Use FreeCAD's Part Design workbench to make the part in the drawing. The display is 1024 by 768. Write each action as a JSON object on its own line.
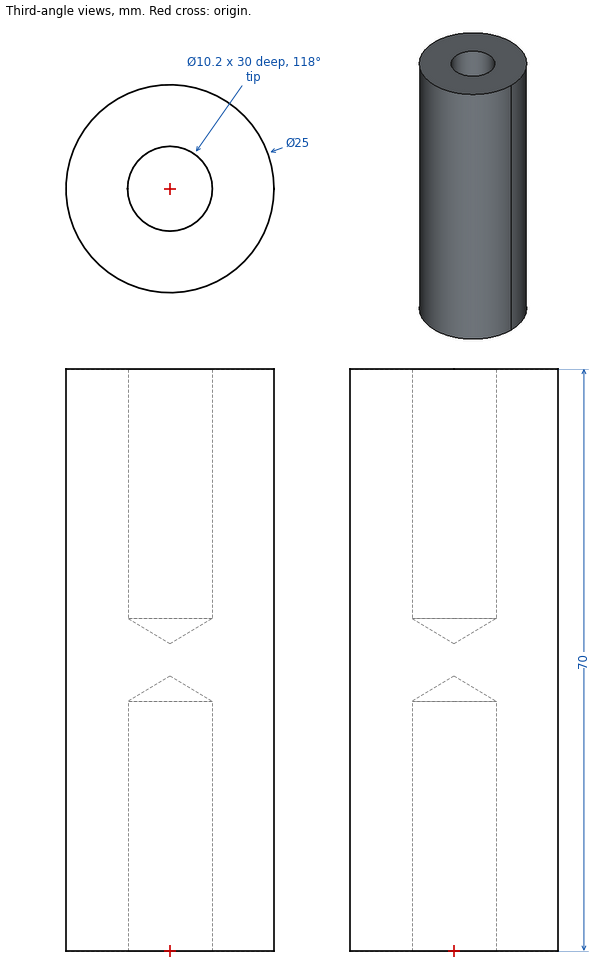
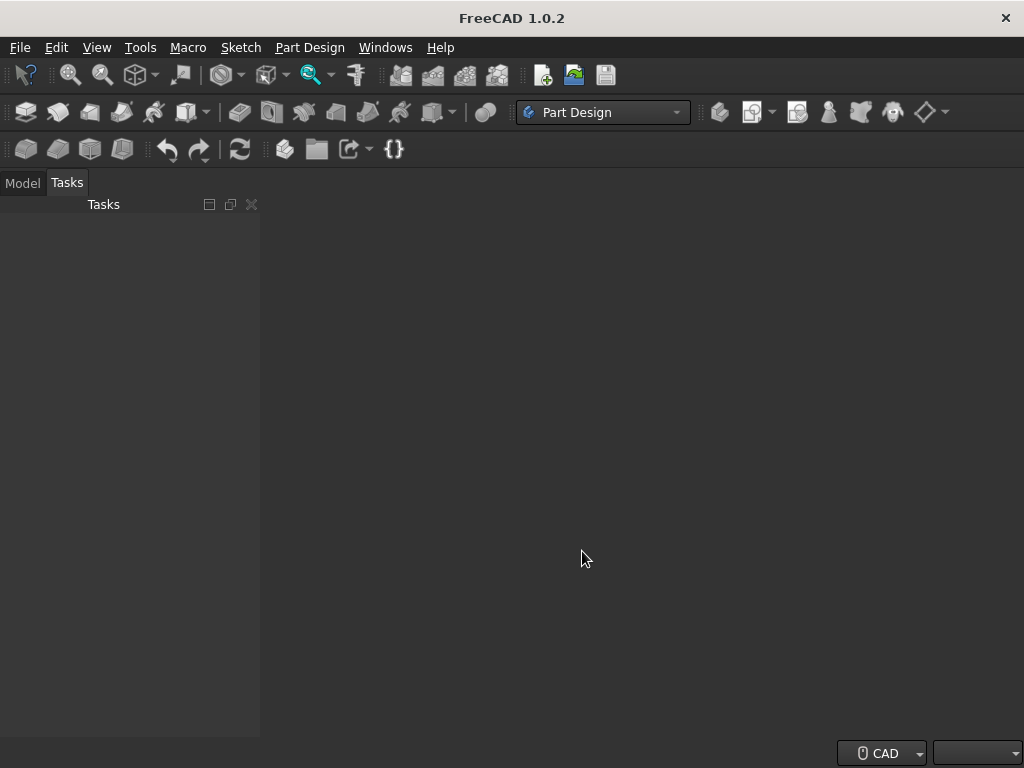
{"action": "key", "text": "ctrl+n"}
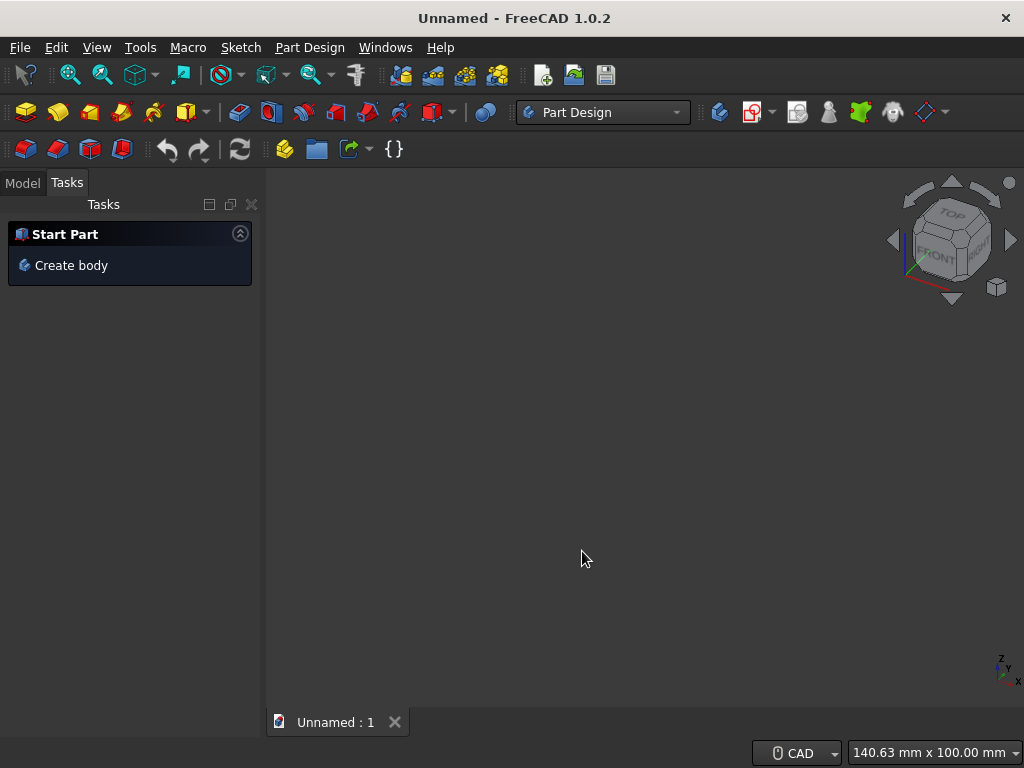
{"action": "left_click", "coordinate": [752, 112]}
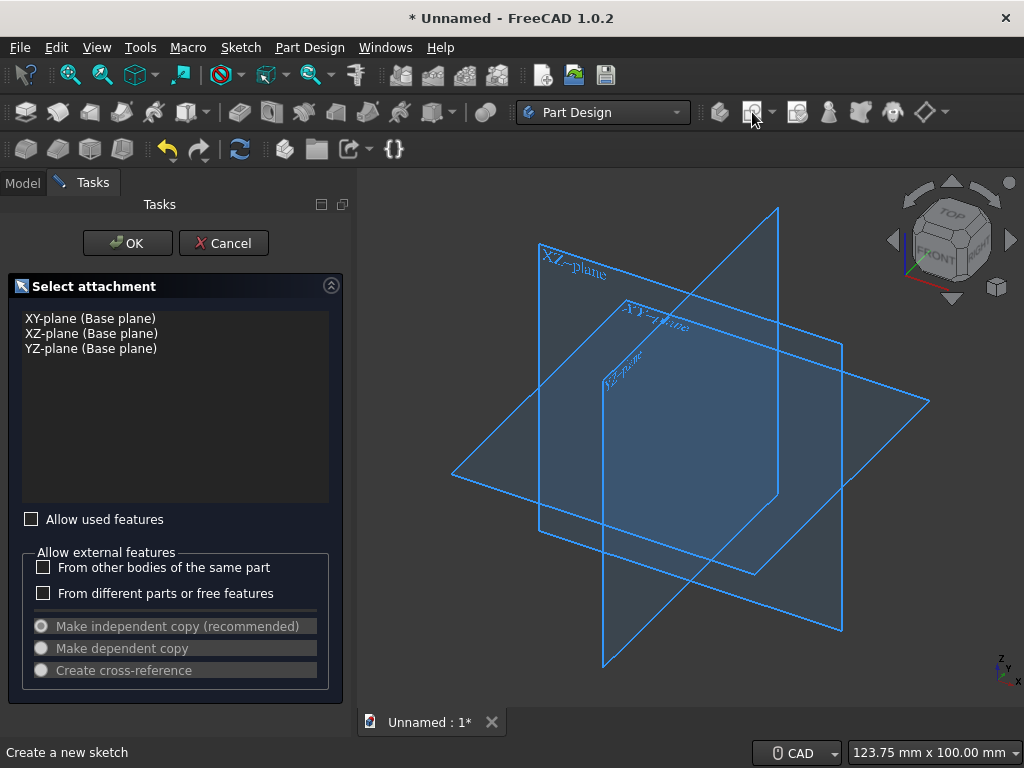
{"action": "left_click", "coordinate": [82, 318]}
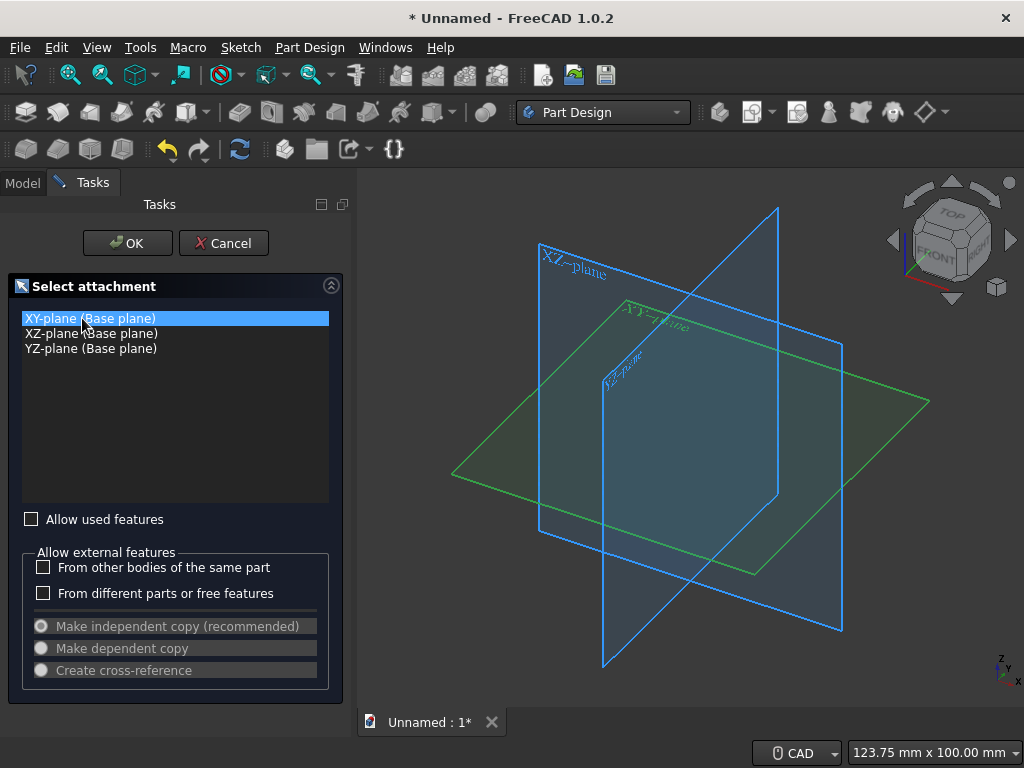
{"action": "left_click", "coordinate": [128, 243]}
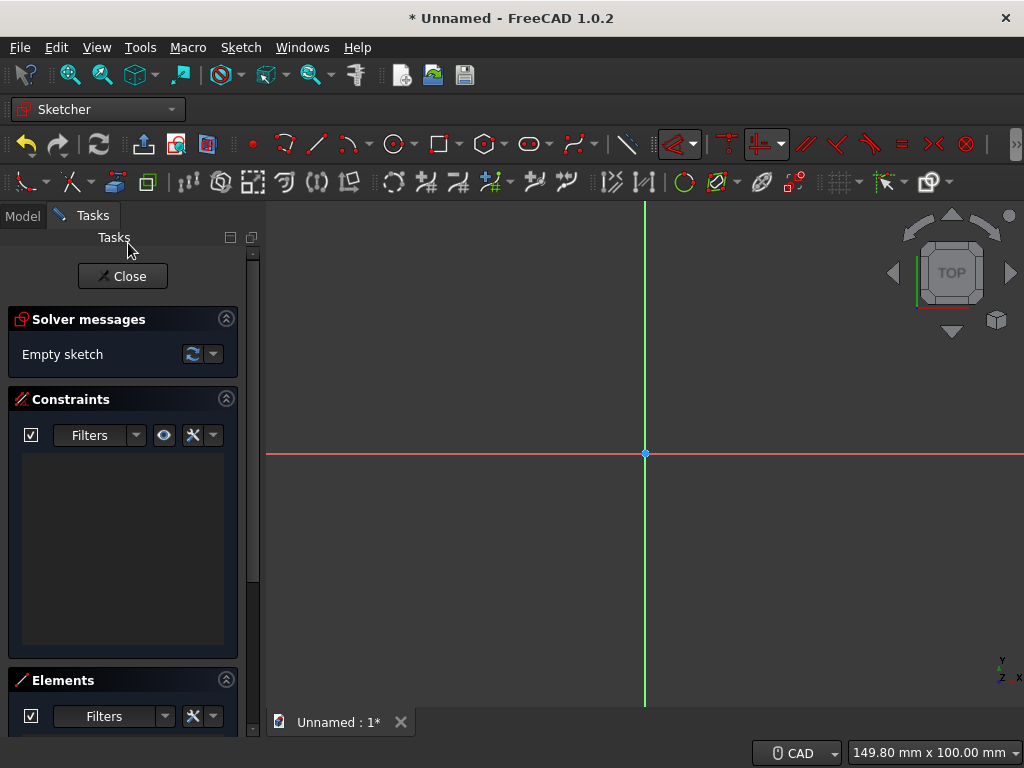
{"action": "scroll", "coordinate": [685, 454], "scroll_direction": "up", "scroll_amount": 5}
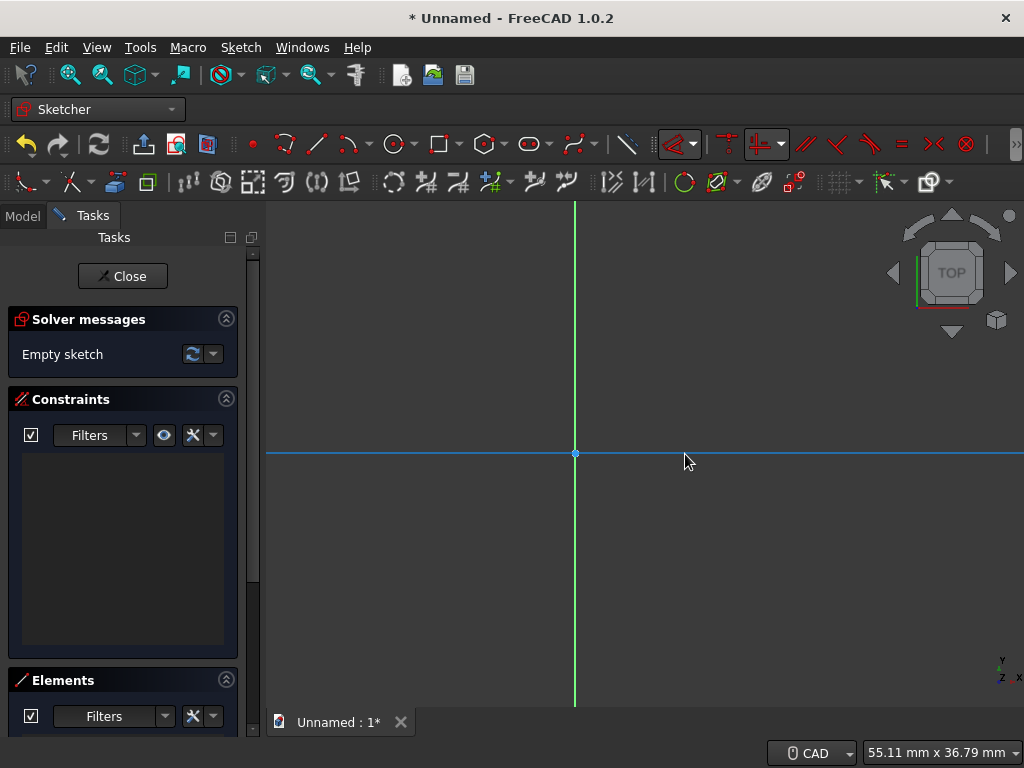
{"action": "key", "text": "g c"}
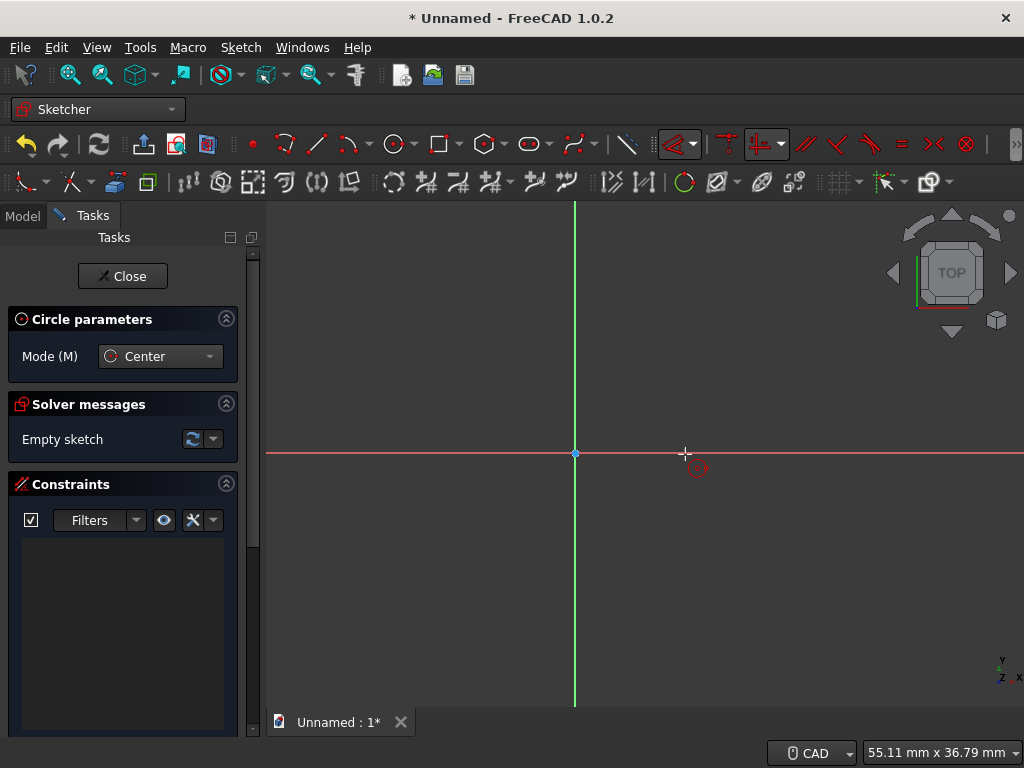
{"action": "left_click", "coordinate": [575, 453]}
{"action": "mouse_move", "coordinate": [697, 332]}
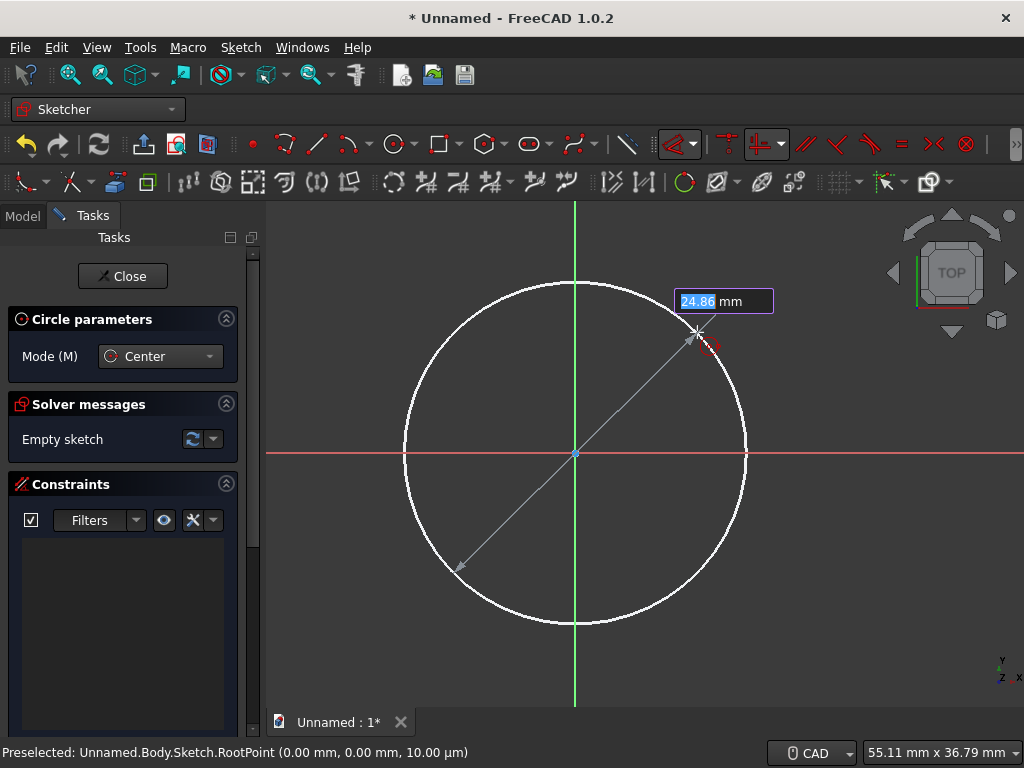
{"action": "type", "text": "25"}
{"action": "key", "text": "Return"}
{"action": "key", "text": "Escape"}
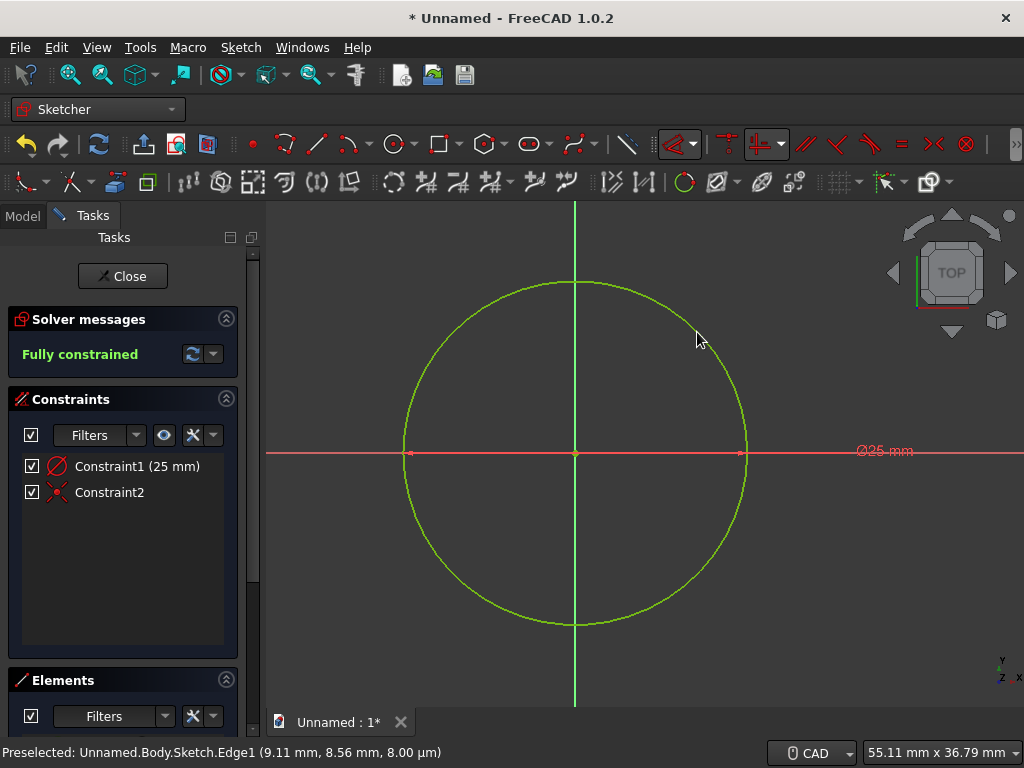
{"action": "left_click", "coordinate": [123, 276]}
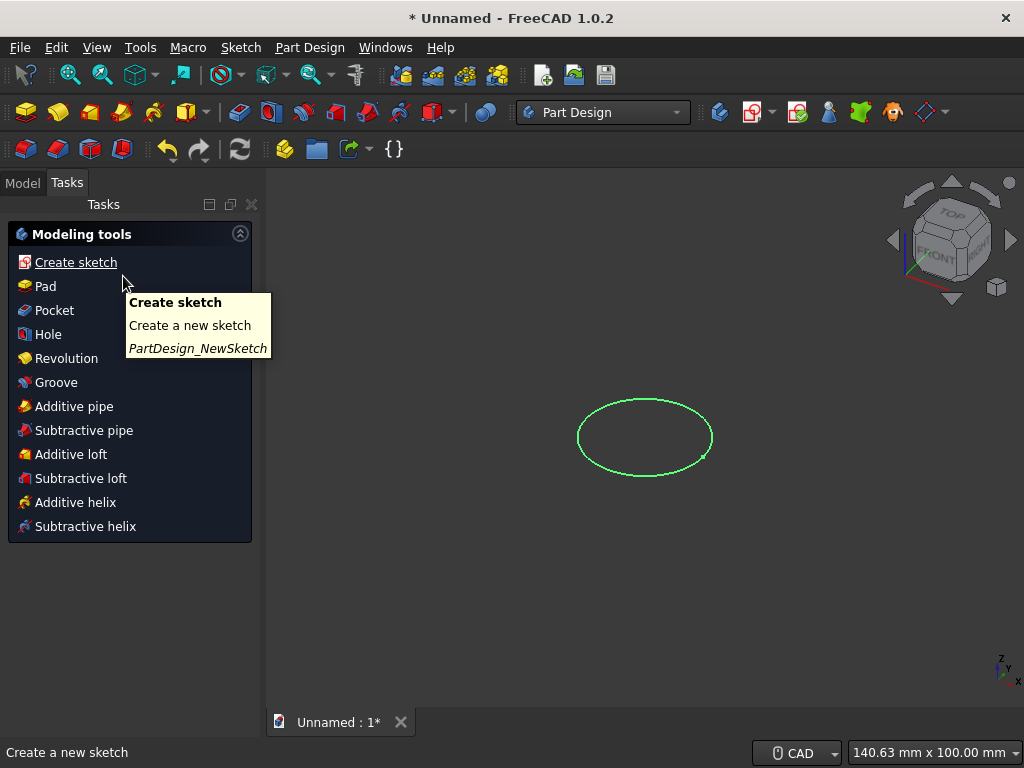
{"action": "left_click", "coordinate": [26, 112]}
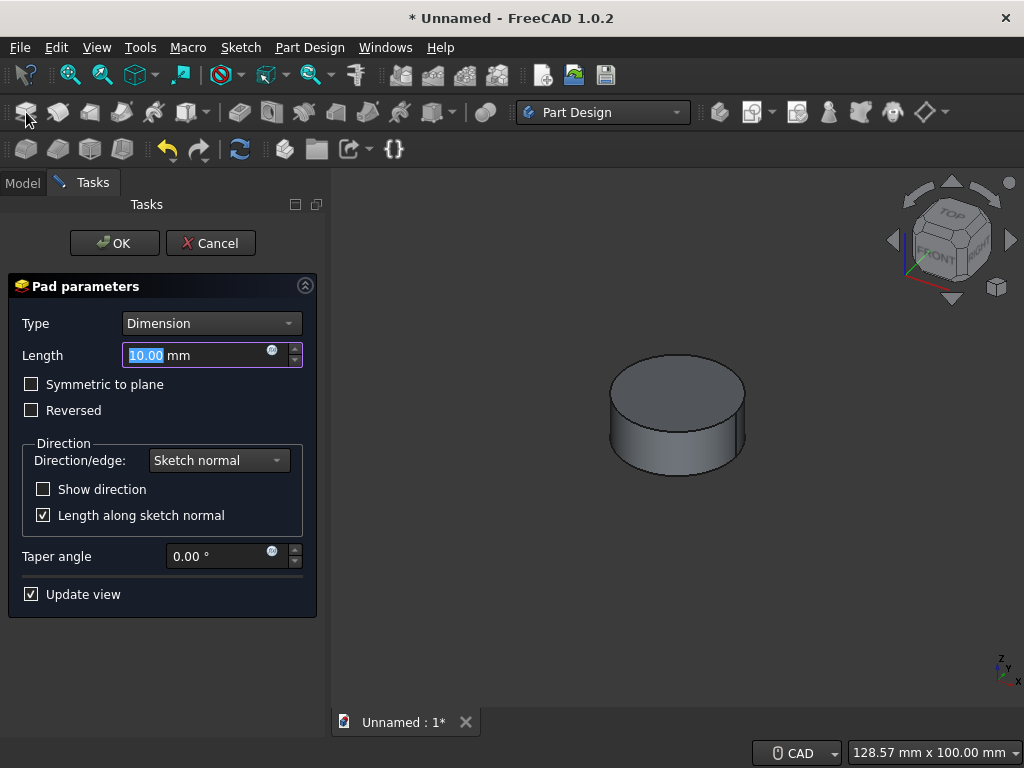
{"action": "type", "text": "70"}
{"action": "key", "text": "Tab"}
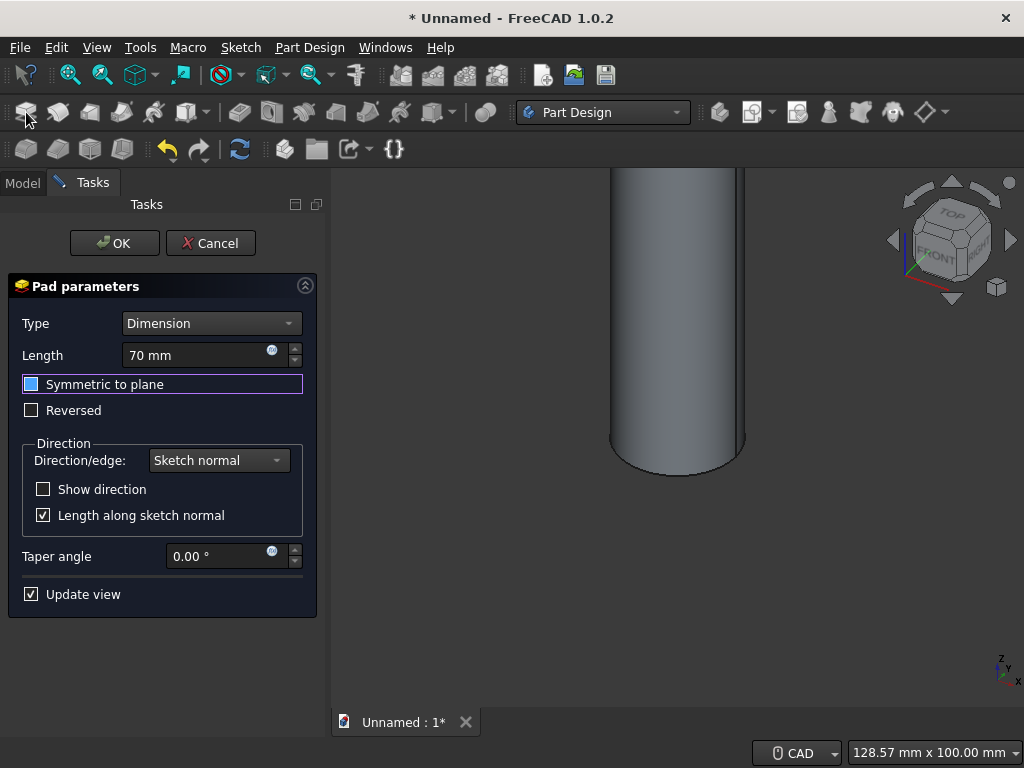
{"action": "left_click", "coordinate": [115, 243]}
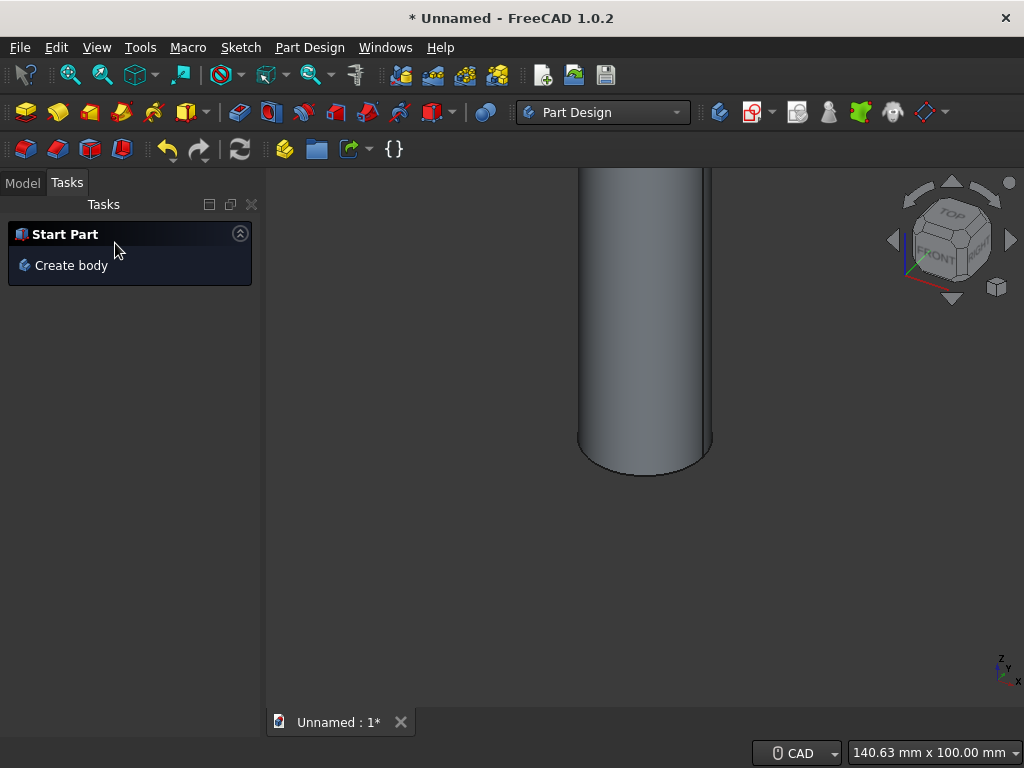
{"action": "left_click", "coordinate": [72, 76]}